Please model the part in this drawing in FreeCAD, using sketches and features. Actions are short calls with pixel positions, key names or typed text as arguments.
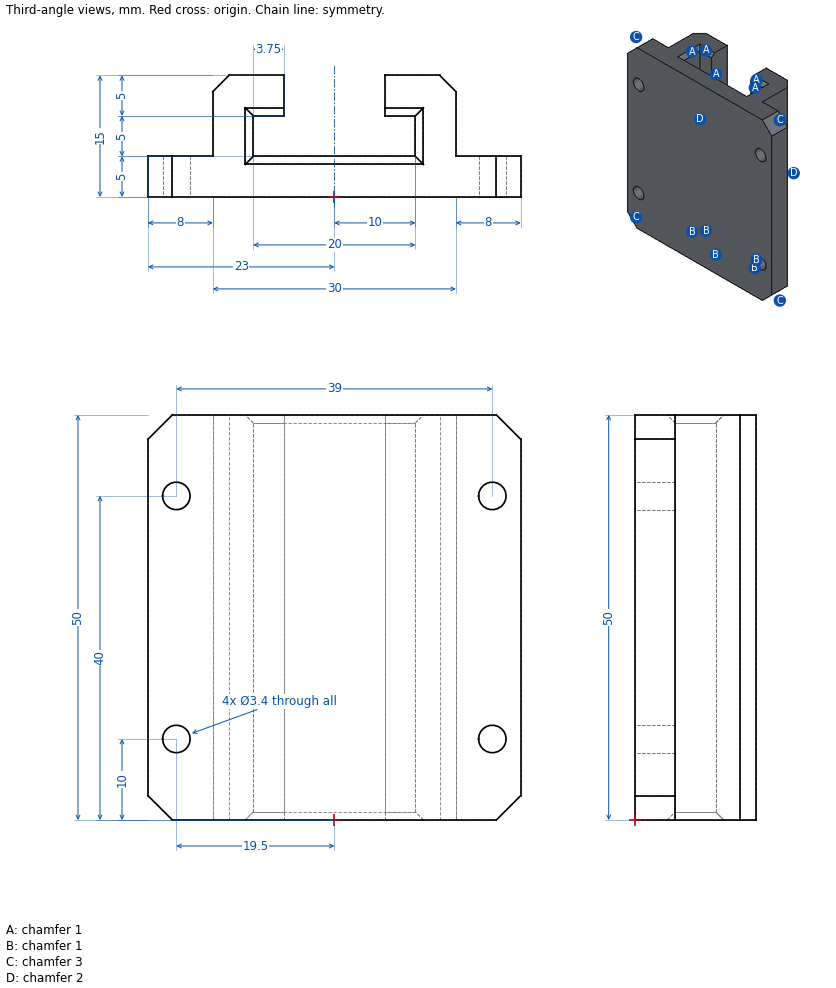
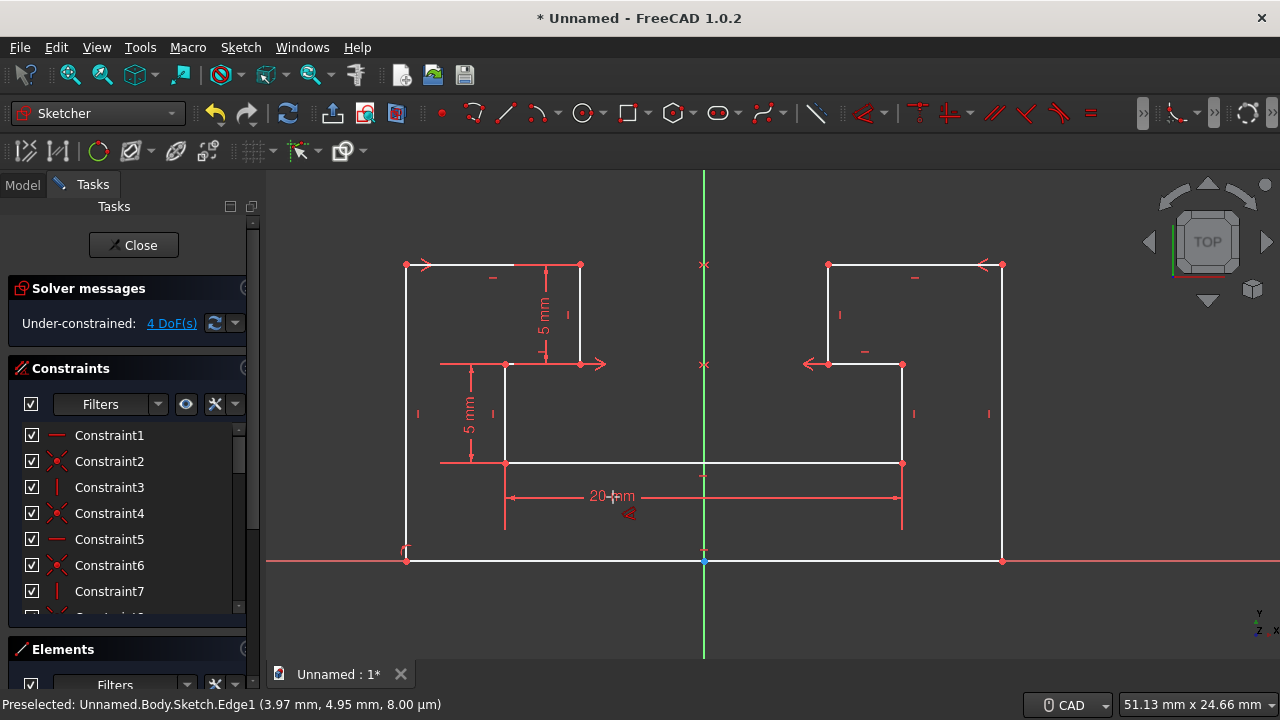
click(406, 354)
click(372, 413)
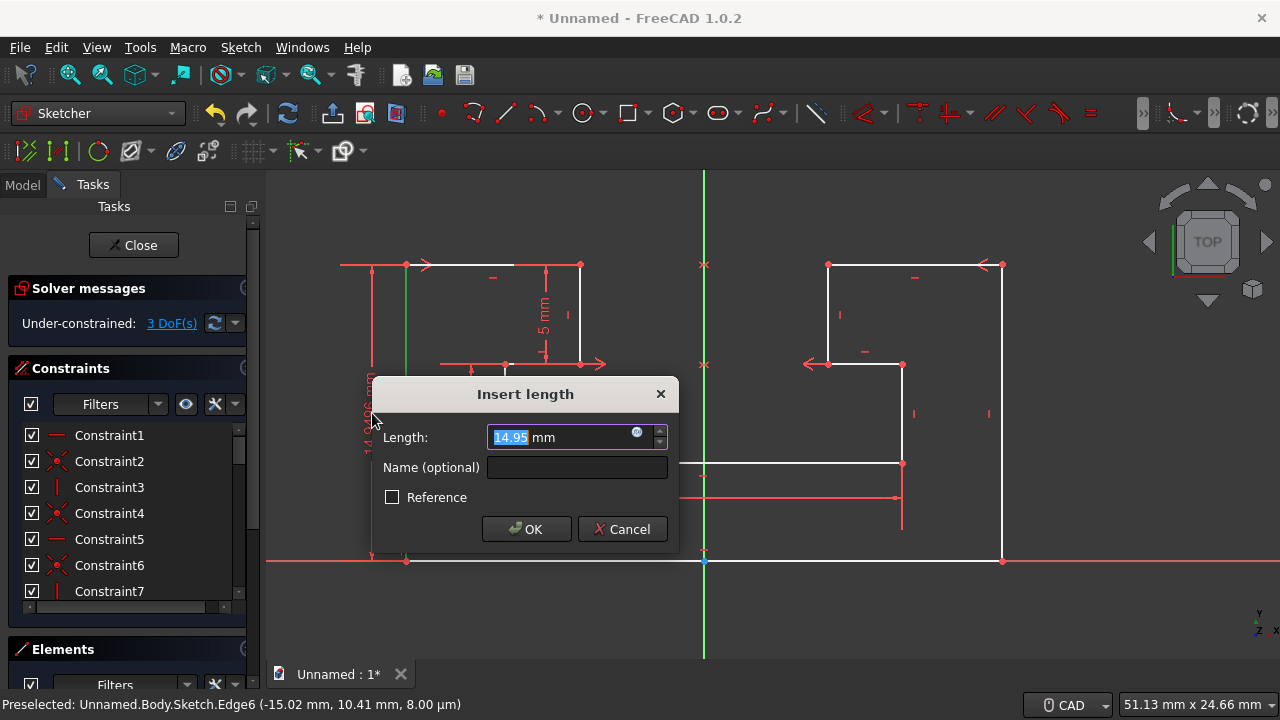
text(15)
key(Return)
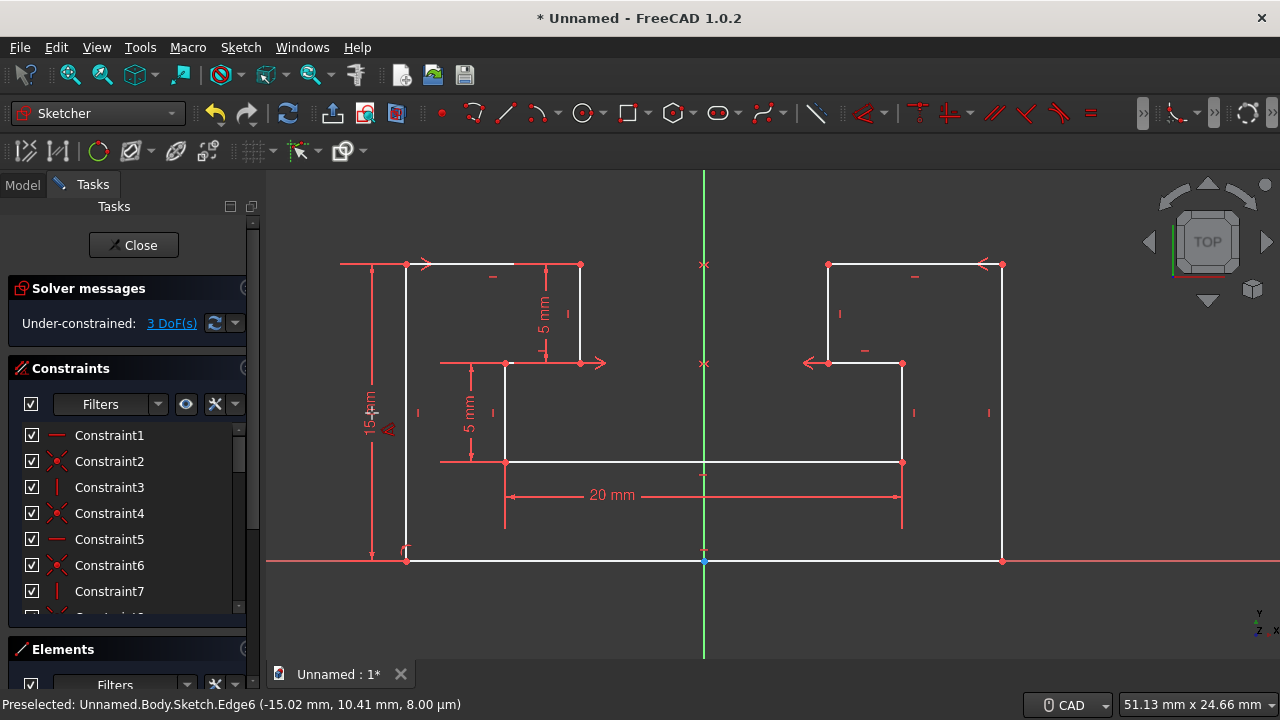
click(585, 561)
click(567, 595)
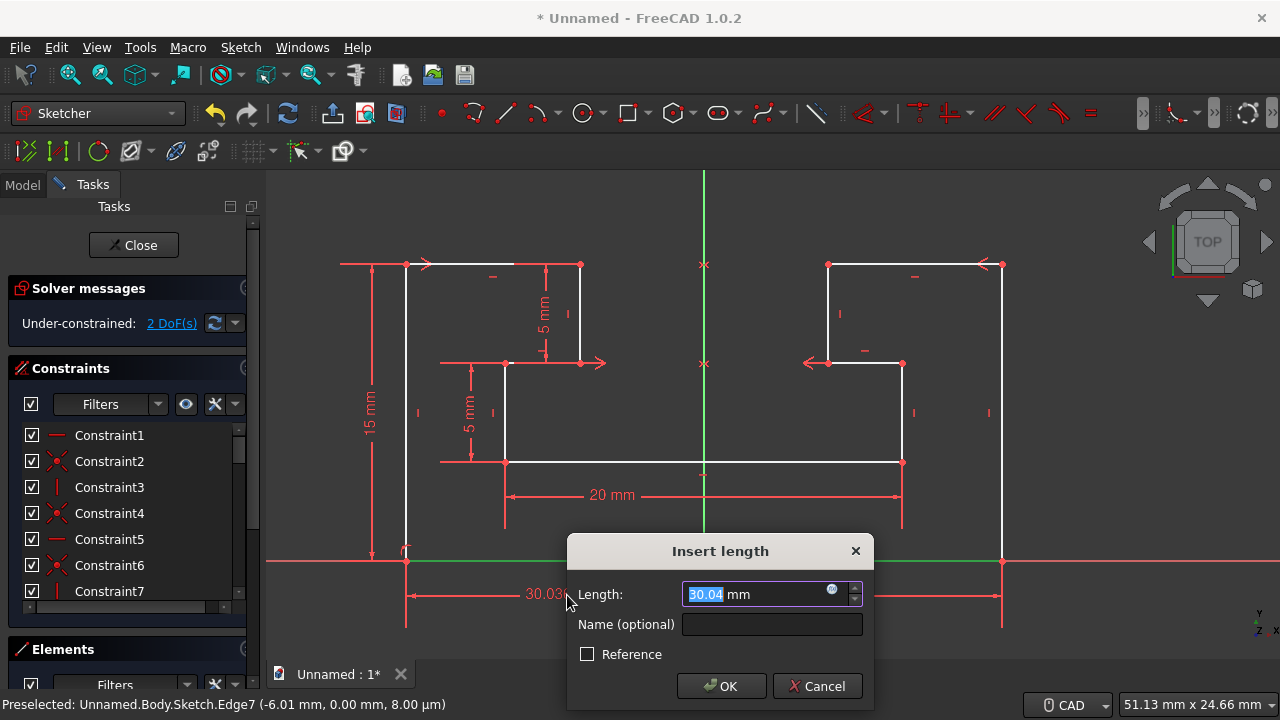
text(30)
key(Return)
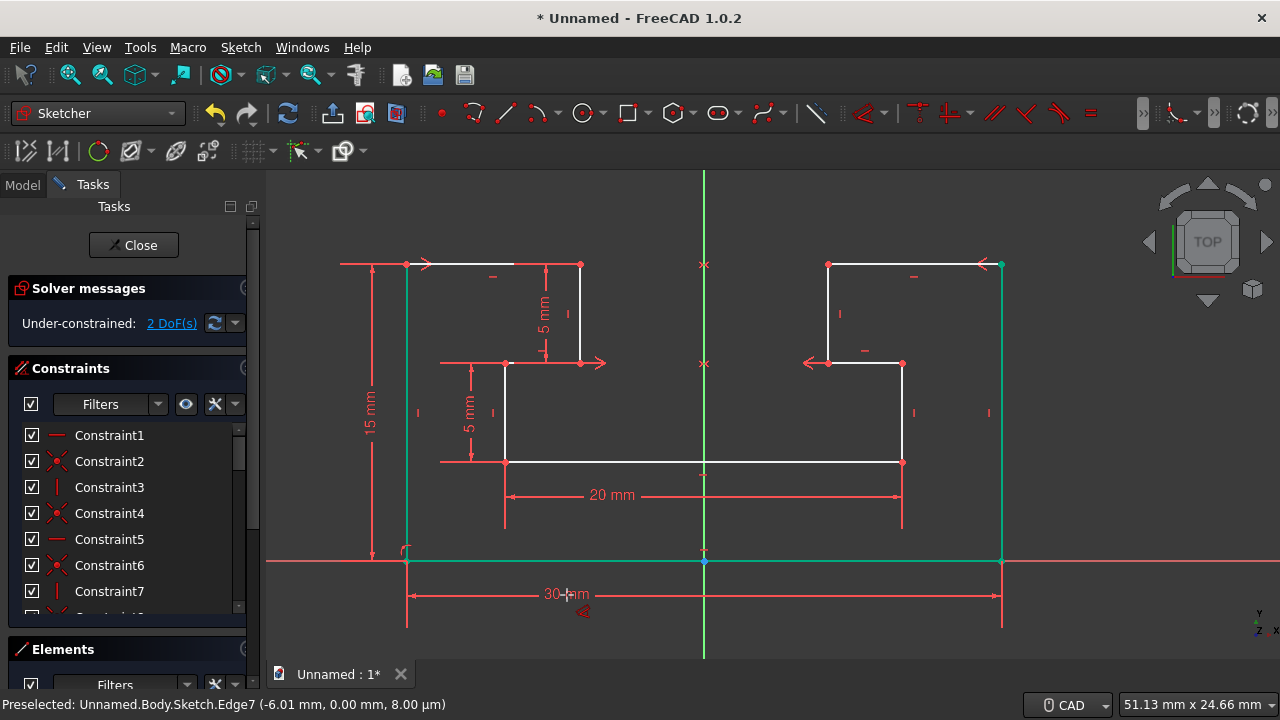
click(902, 462)
click(803, 595)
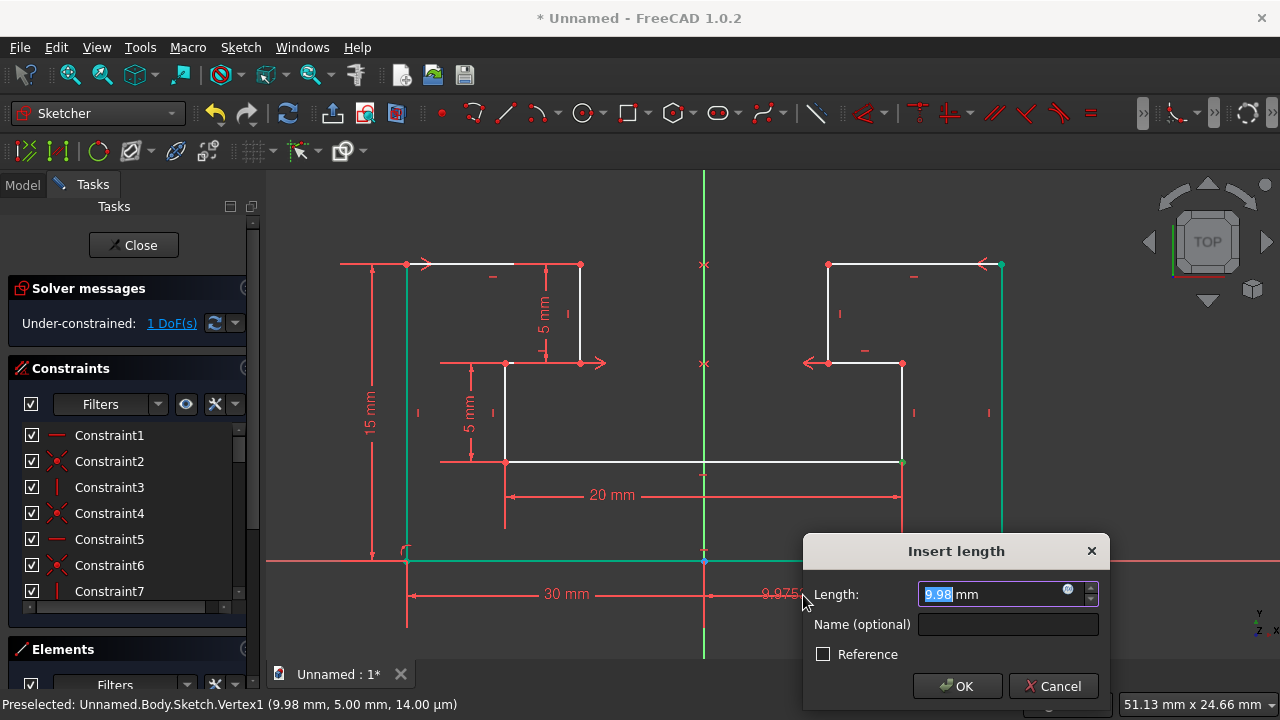
text(10)
key(Return)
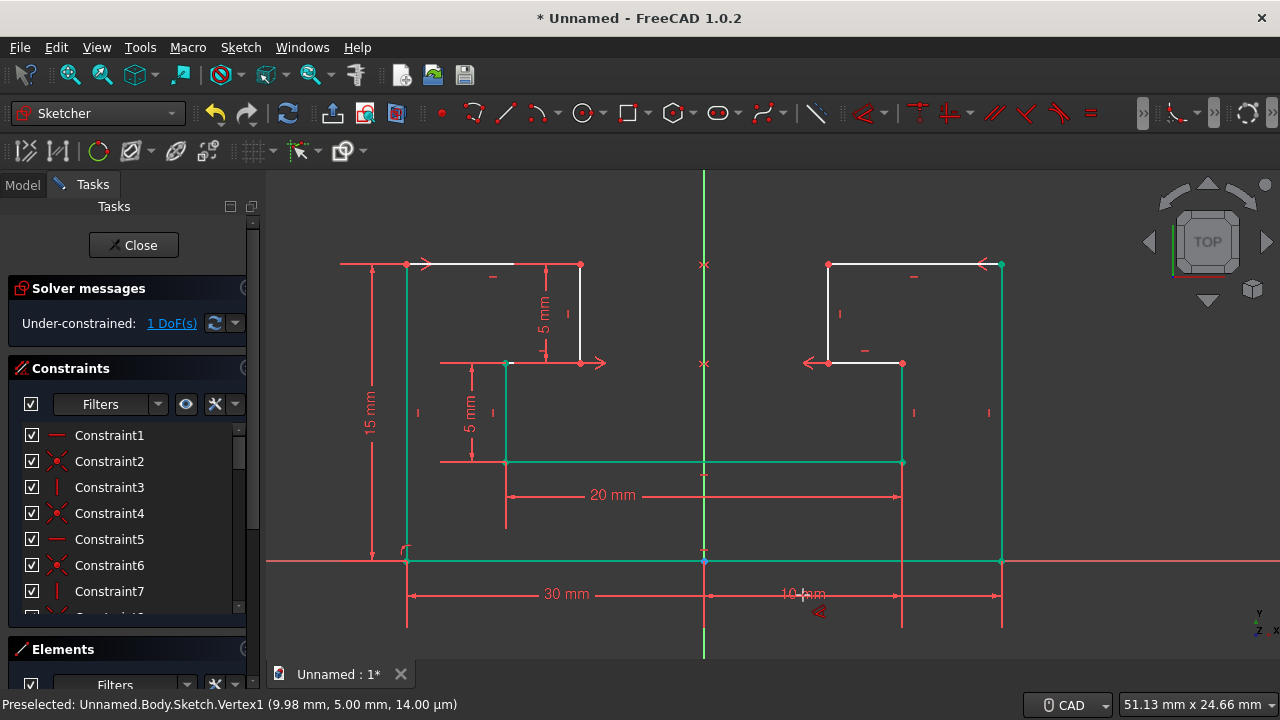
click(528, 363)
click(543, 397)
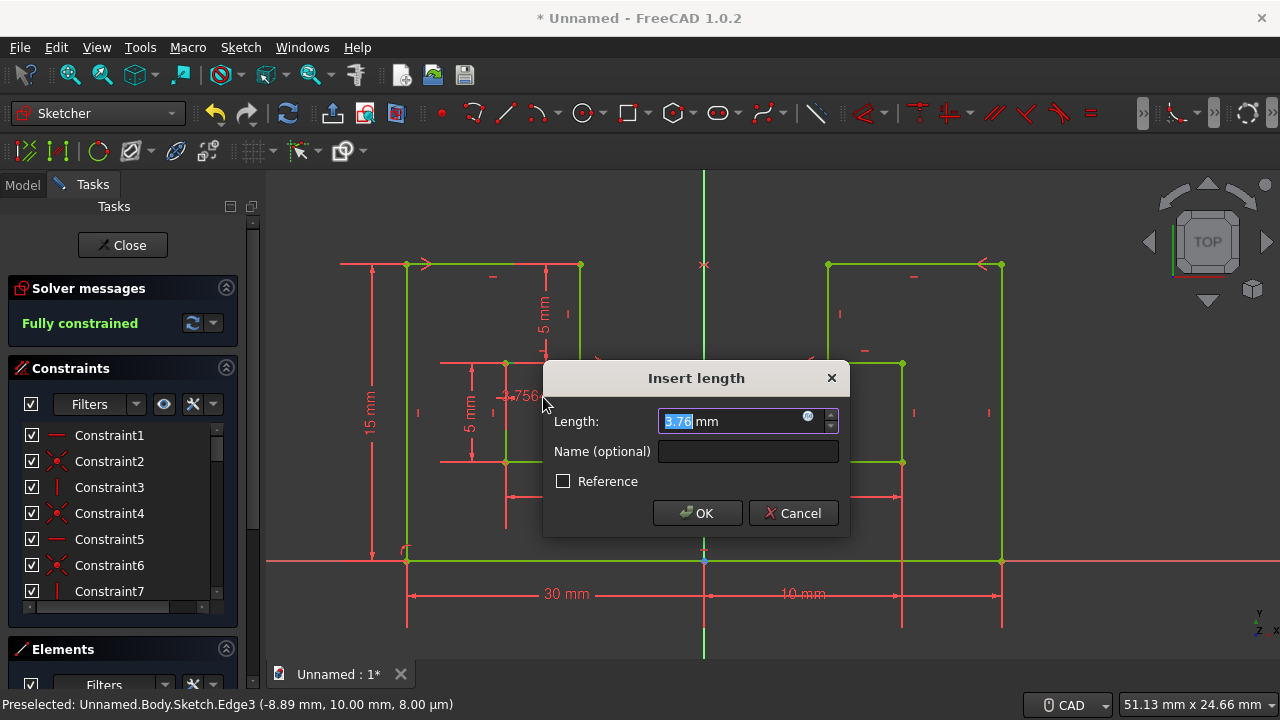
text(3.75)
key(Return)
key(Escape)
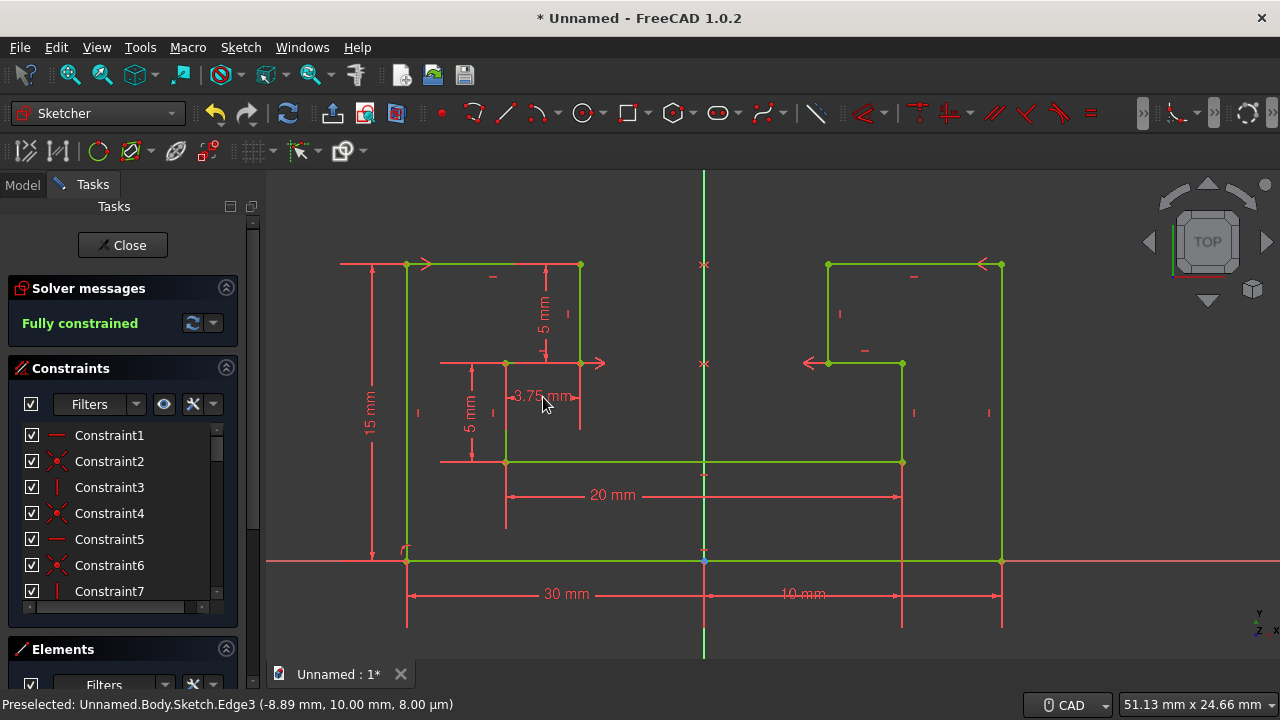
click(123, 245)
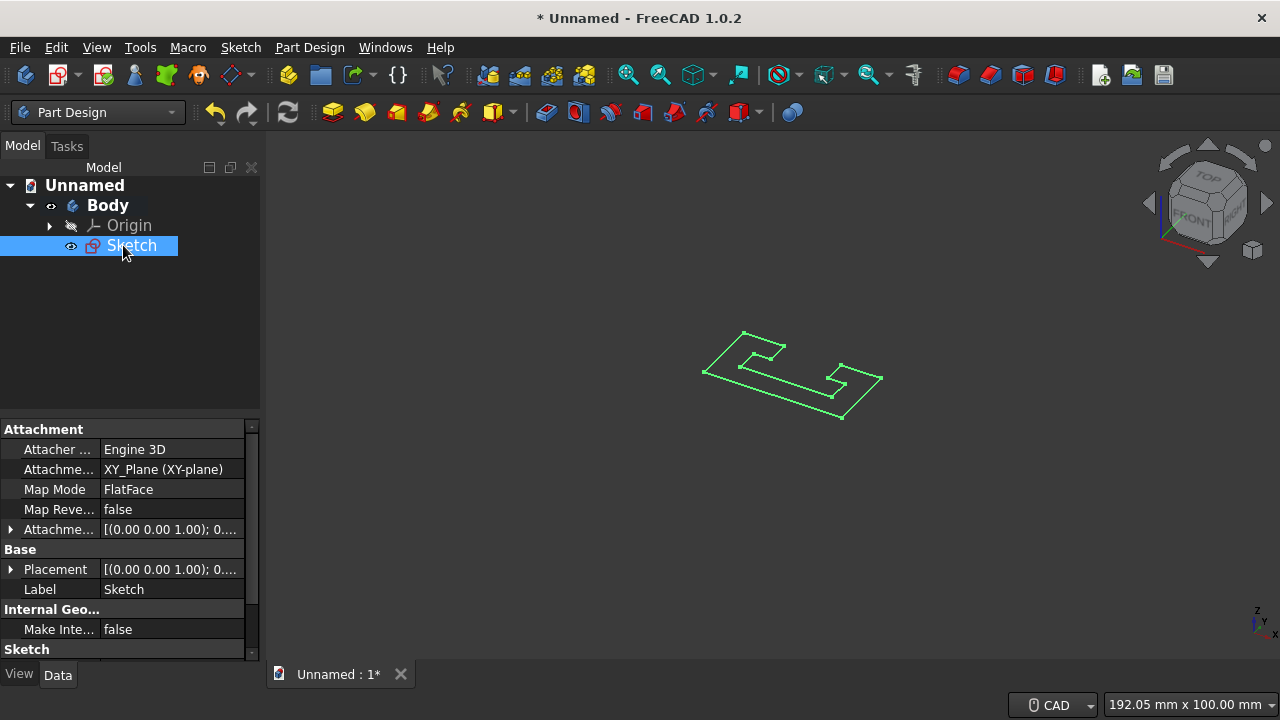
click(334, 112)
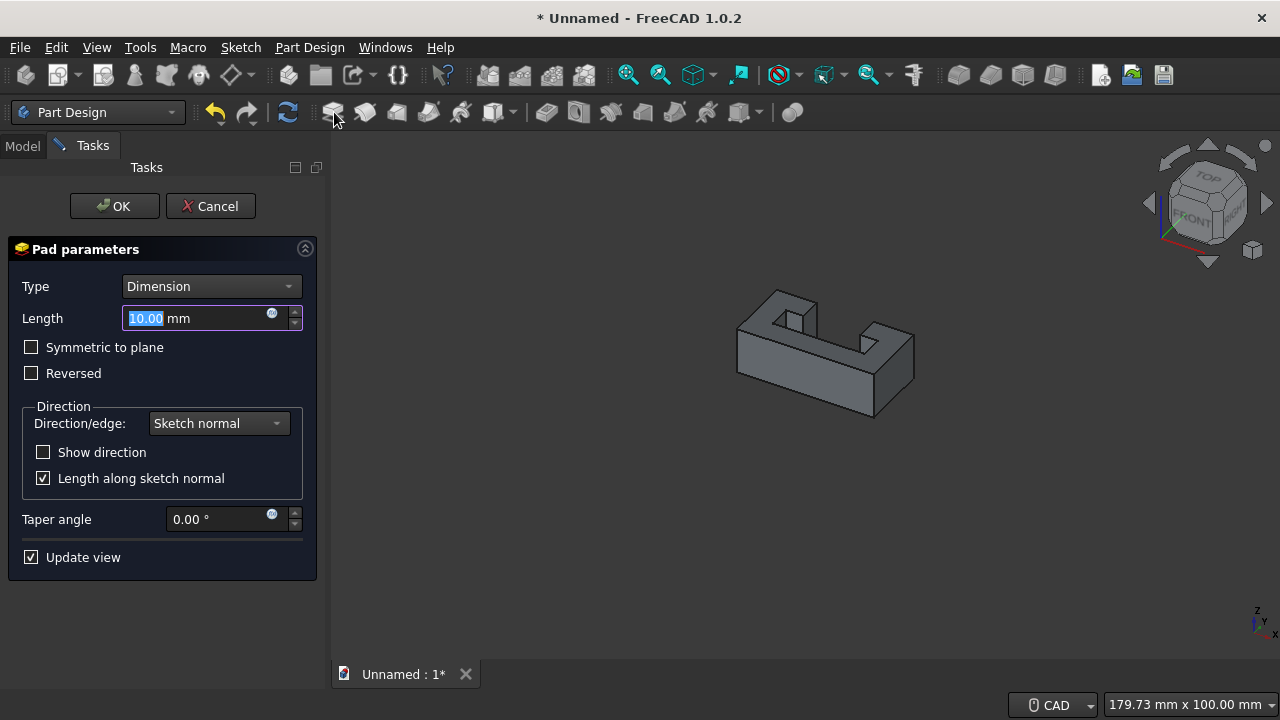
text(50)
key(Tab)